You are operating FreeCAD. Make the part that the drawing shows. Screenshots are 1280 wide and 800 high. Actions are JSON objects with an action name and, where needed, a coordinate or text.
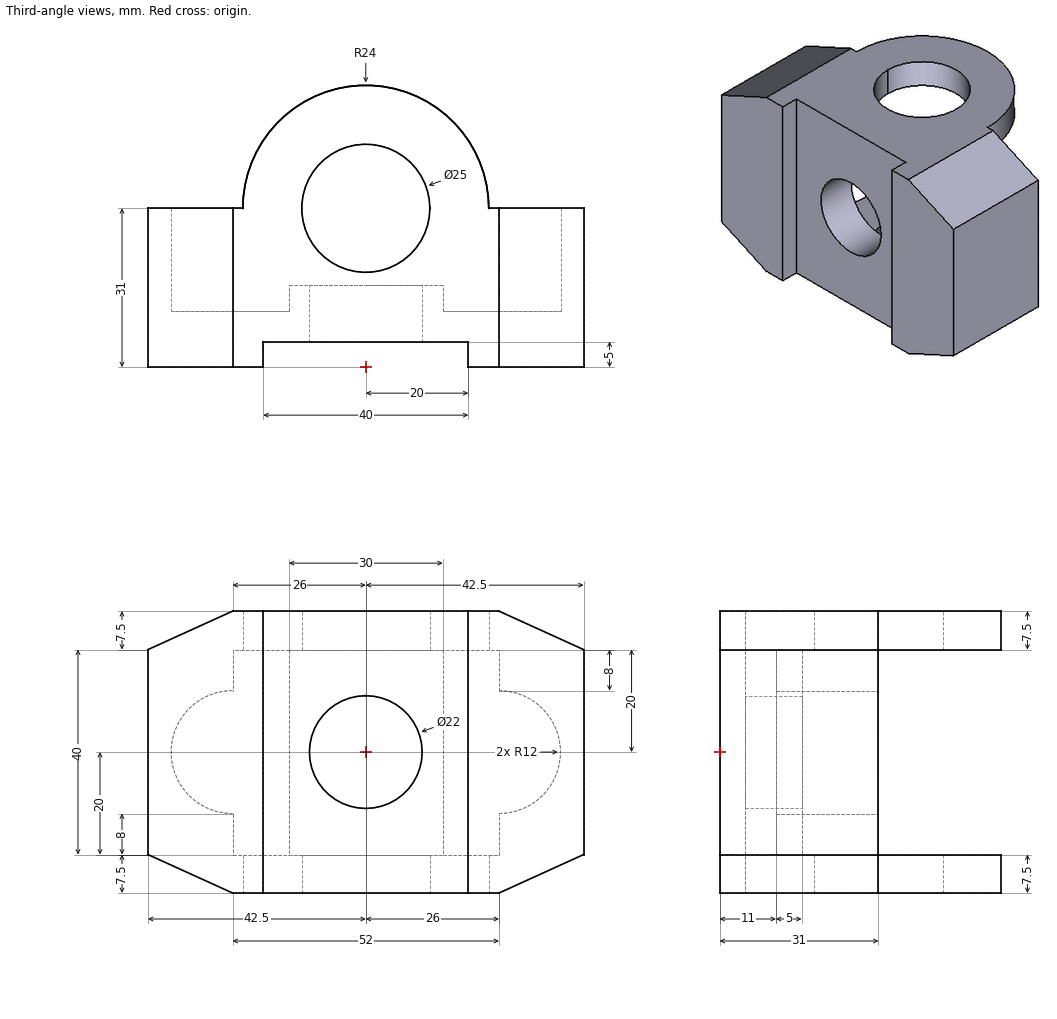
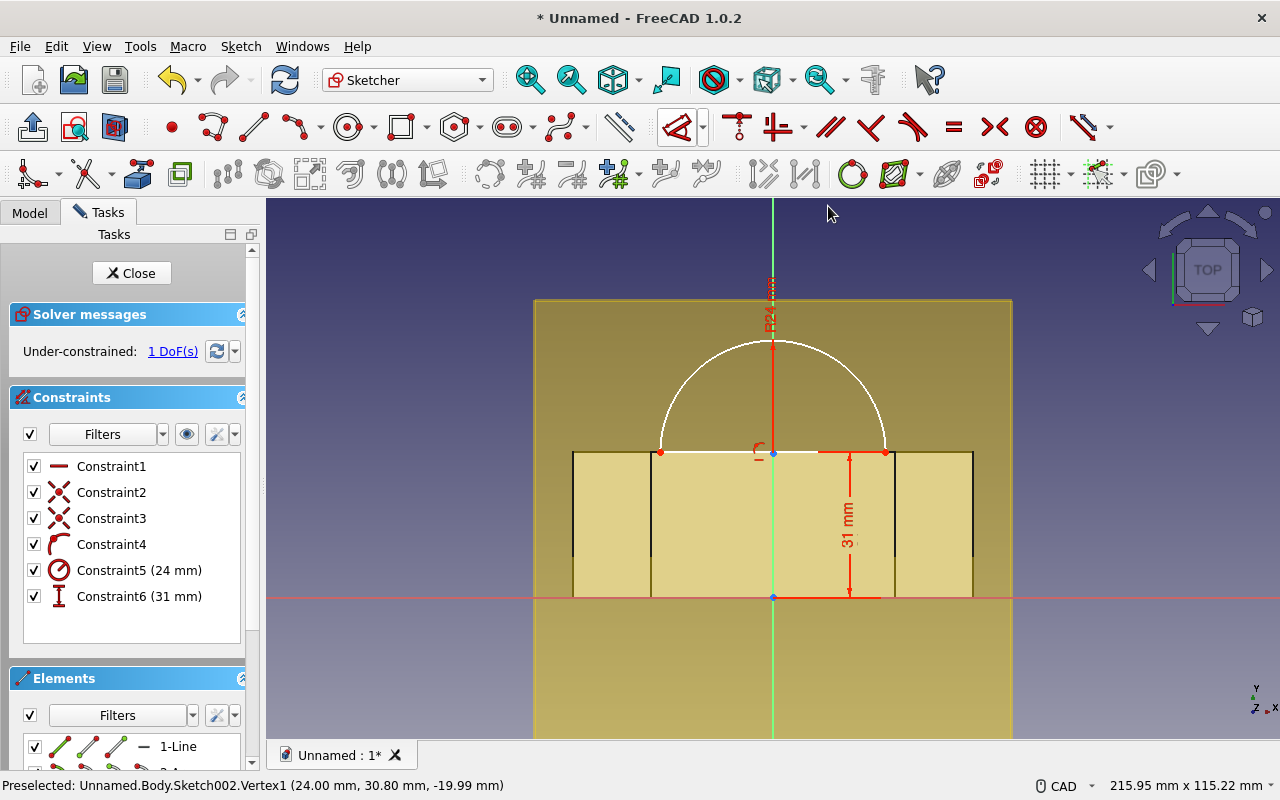
{"action": "left_click", "coordinate": [773, 453]}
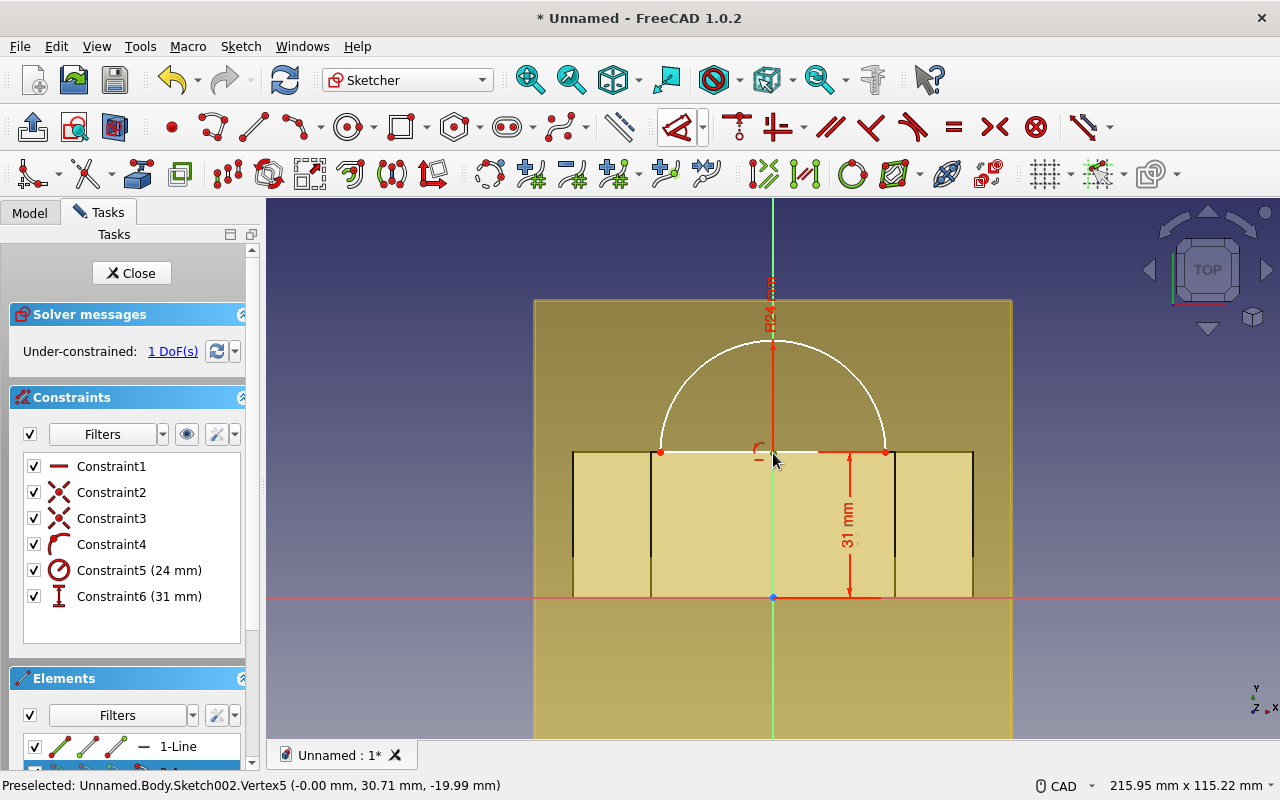
{"action": "left_click", "coordinate": [702, 128]}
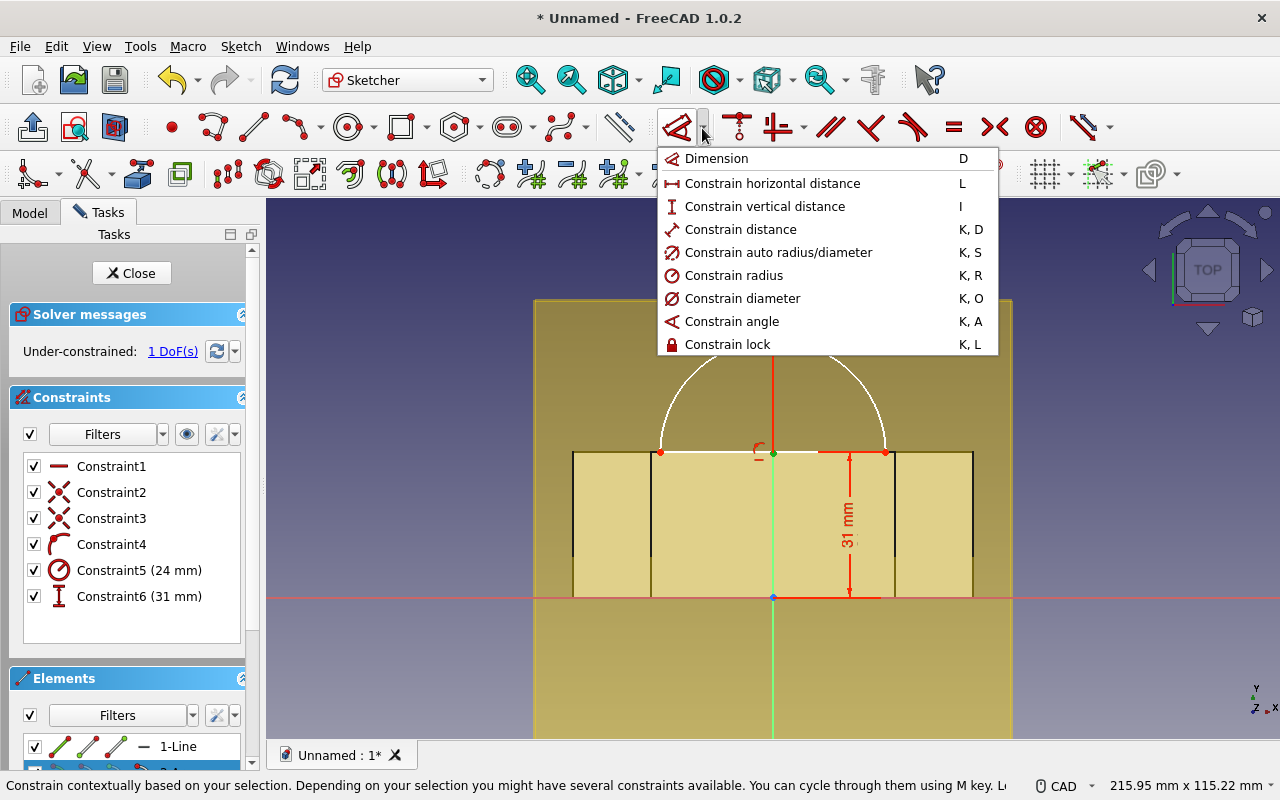
{"action": "left_click", "coordinate": [828, 206]}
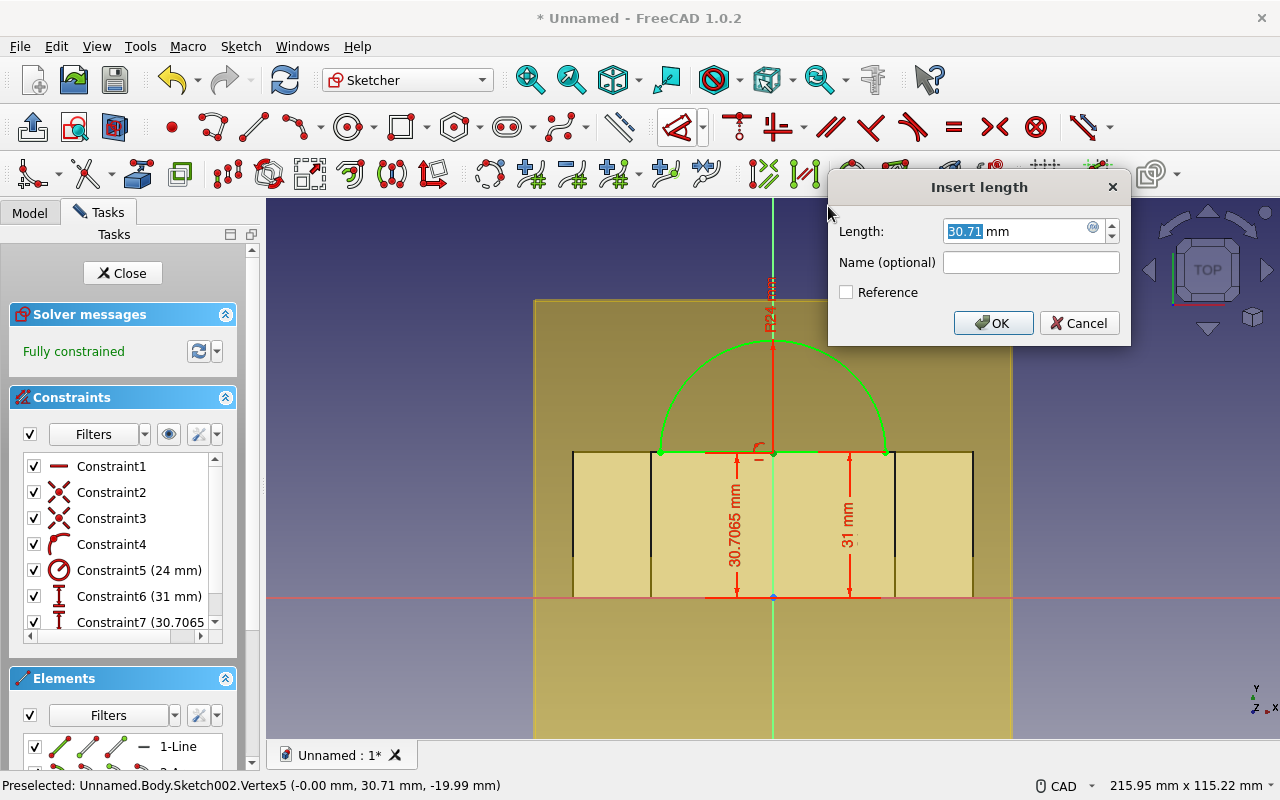
{"action": "type", "text": "31"}
{"action": "key", "text": "Return"}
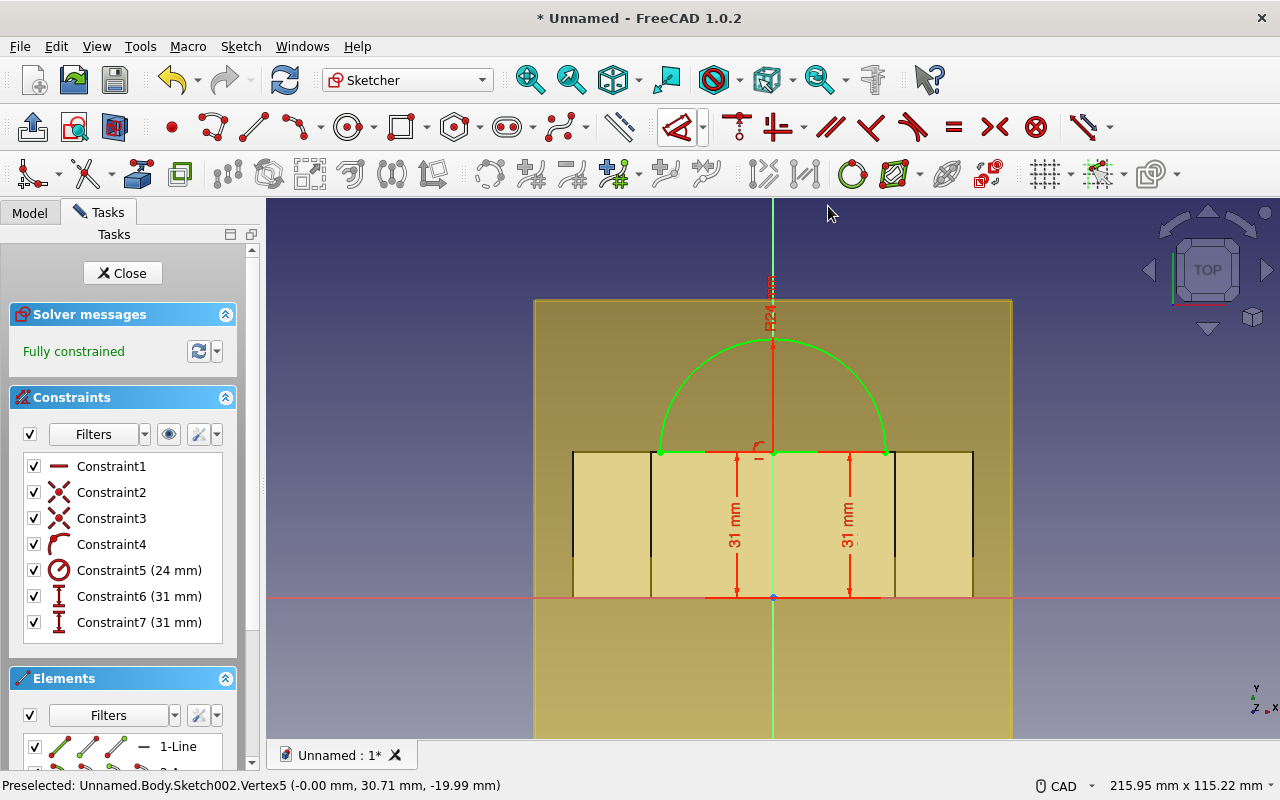
{"action": "left_click", "coordinate": [123, 273]}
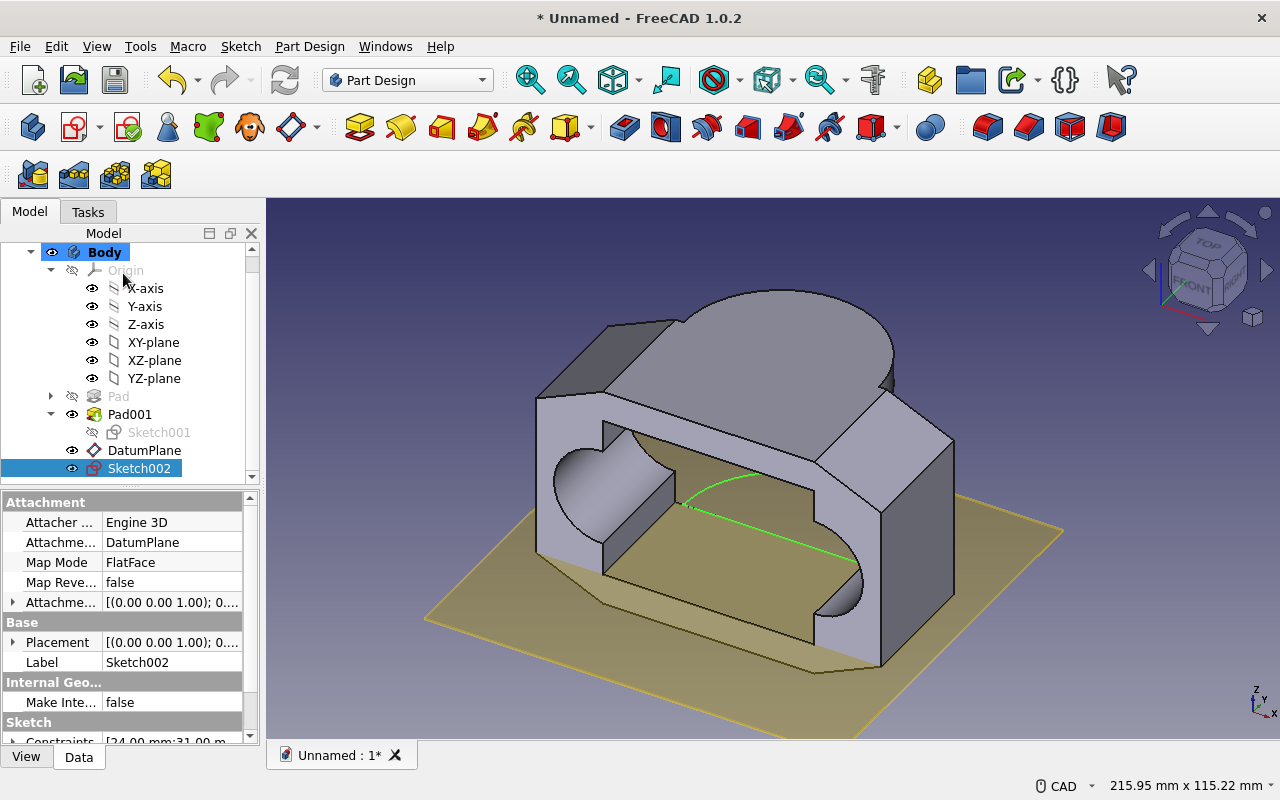
{"action": "left_click", "coordinate": [360, 128]}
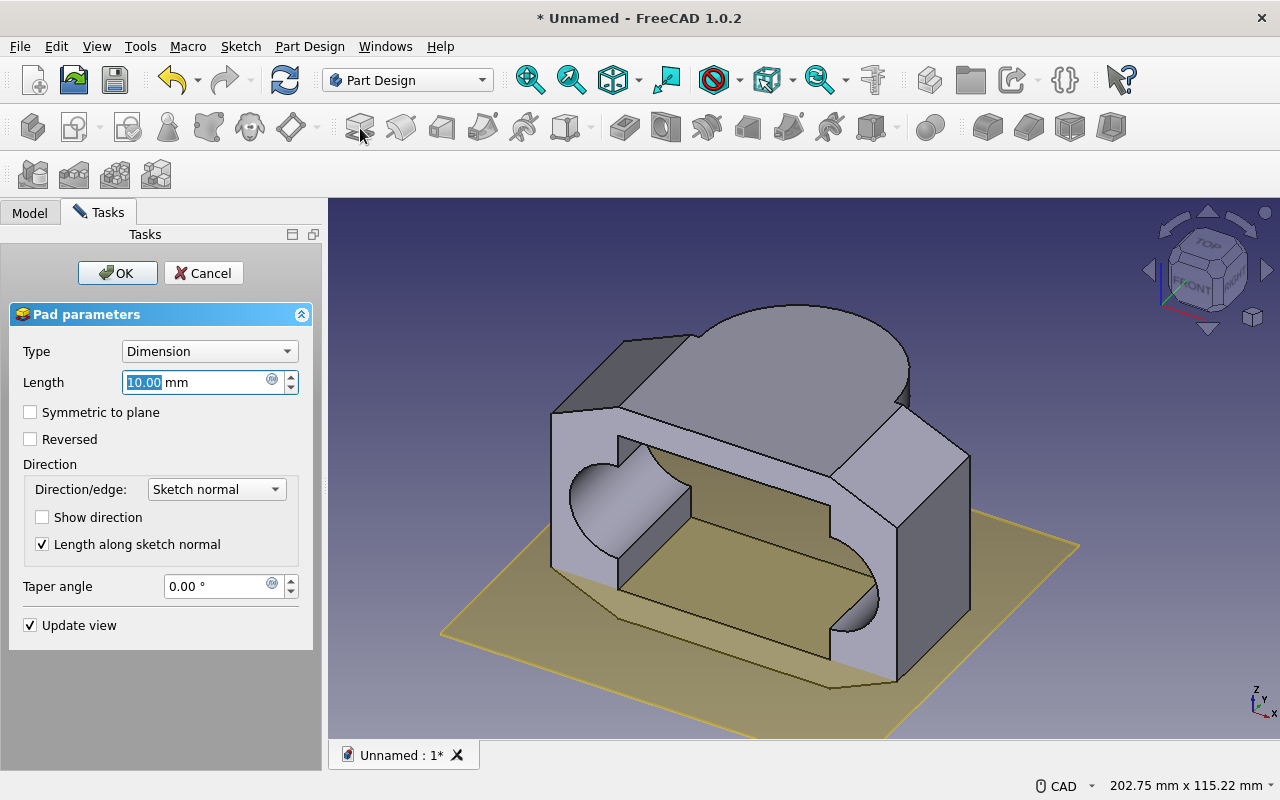
{"action": "type", "text": "7.5"}
{"action": "key", "text": "Tab"}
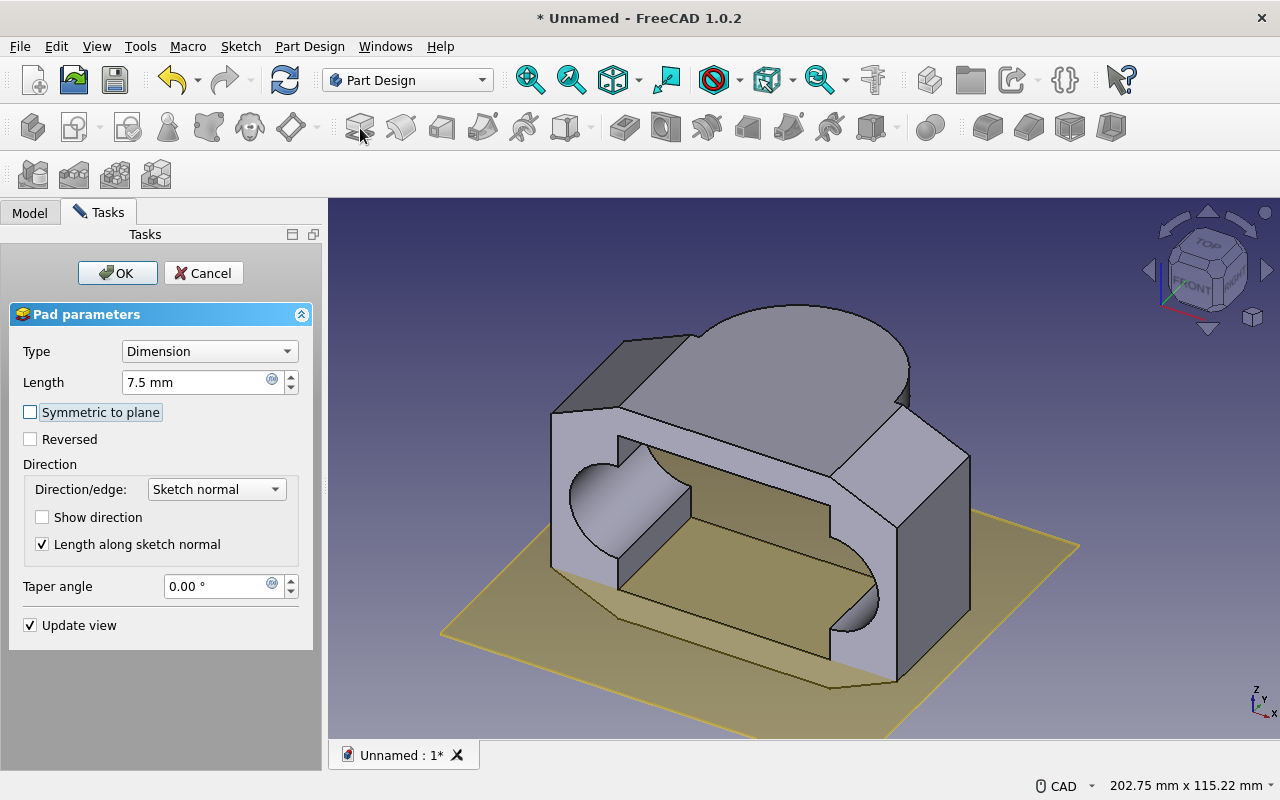
{"action": "left_click", "coordinate": [31, 439]}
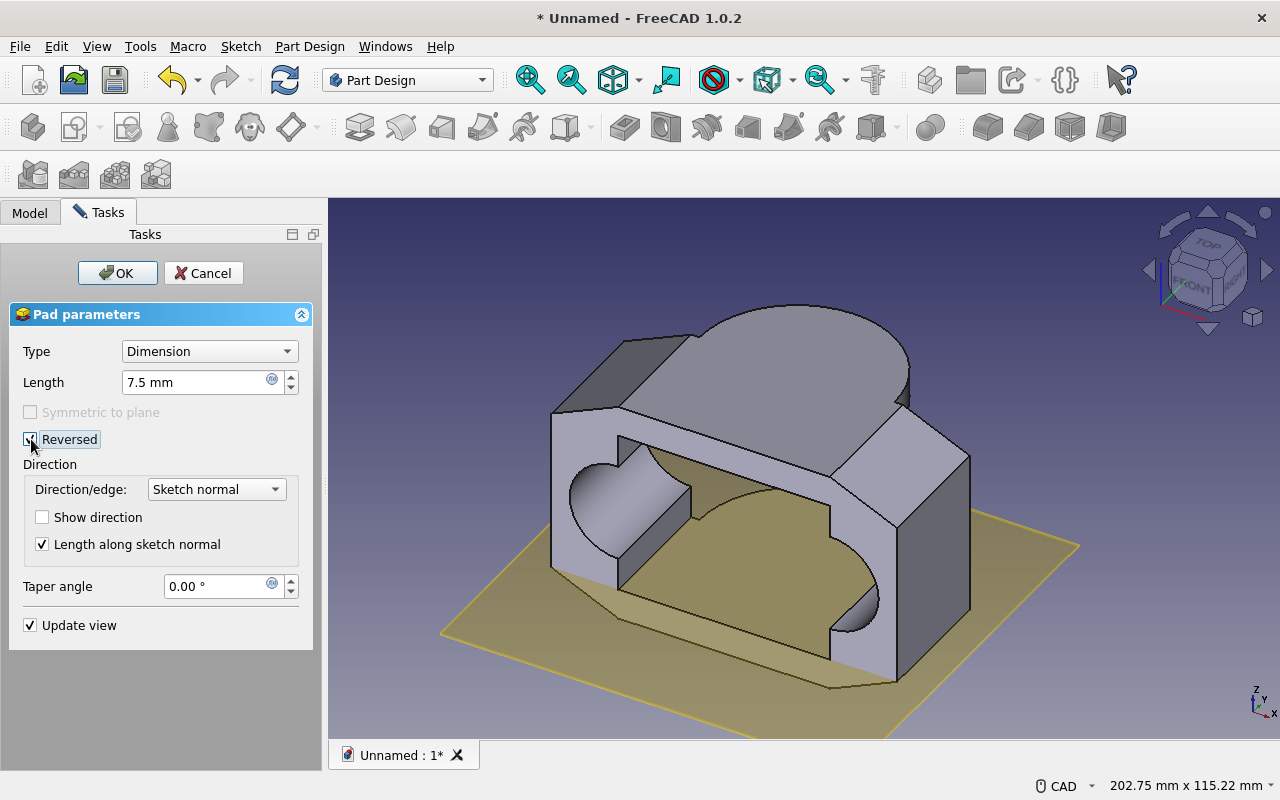
{"action": "left_click", "coordinate": [118, 273]}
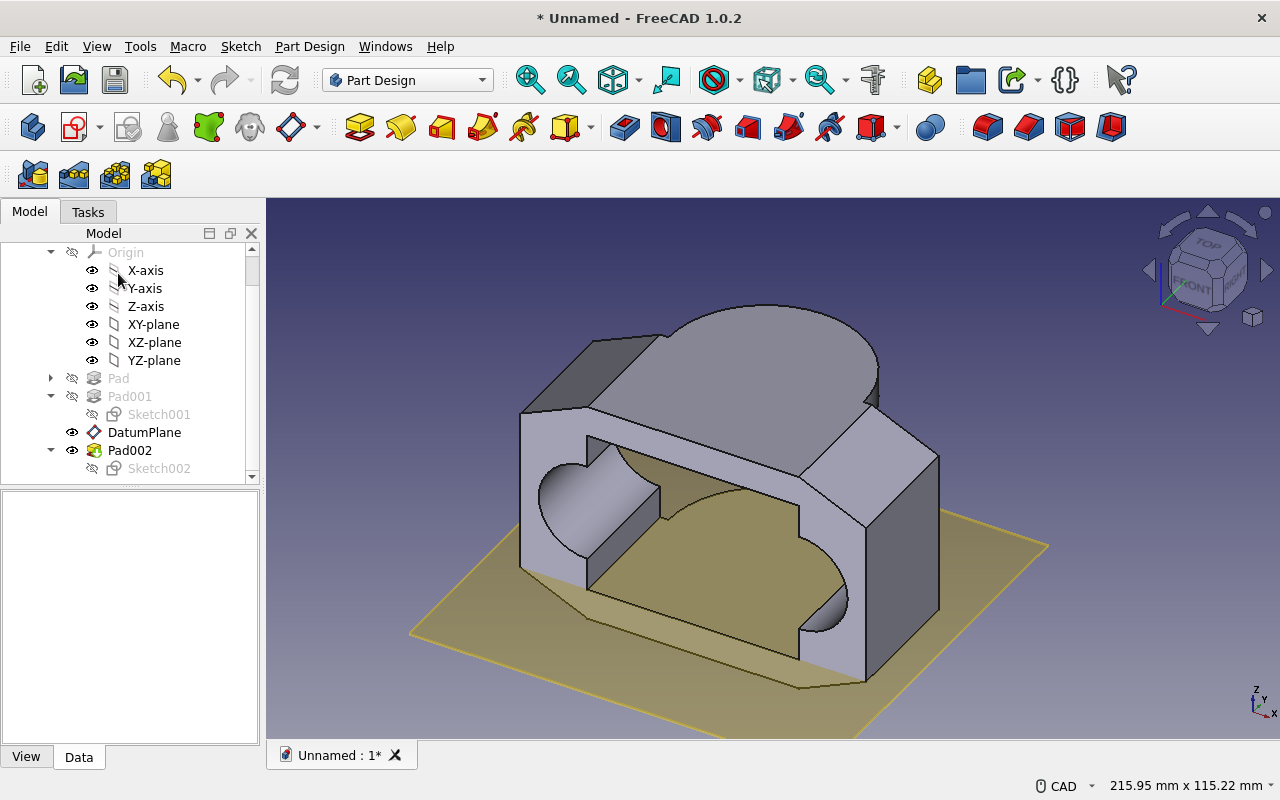
{"action": "left_click", "coordinate": [117, 432]}
{"action": "key", "text": "space"}